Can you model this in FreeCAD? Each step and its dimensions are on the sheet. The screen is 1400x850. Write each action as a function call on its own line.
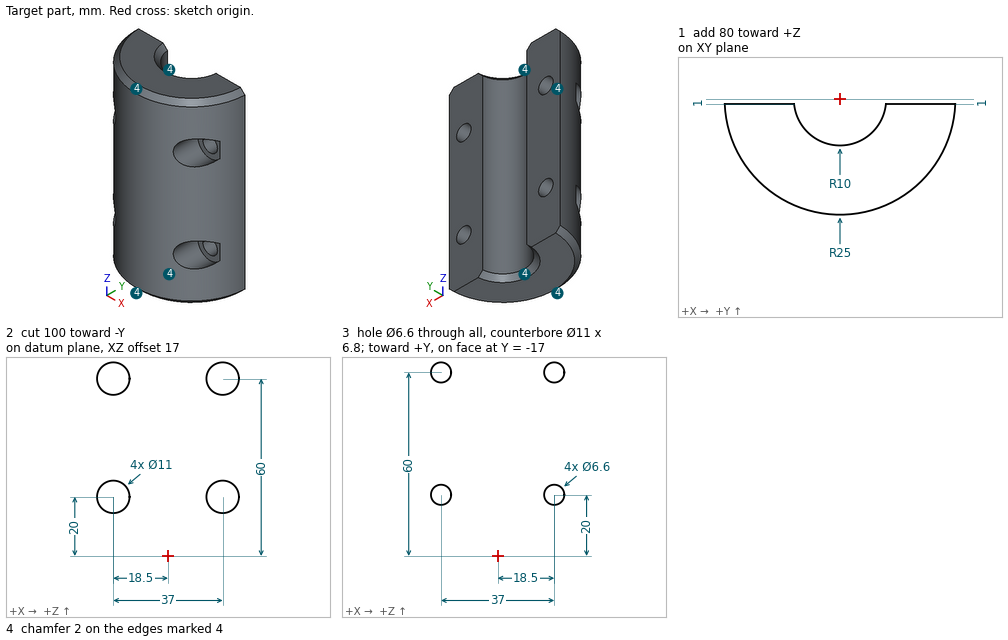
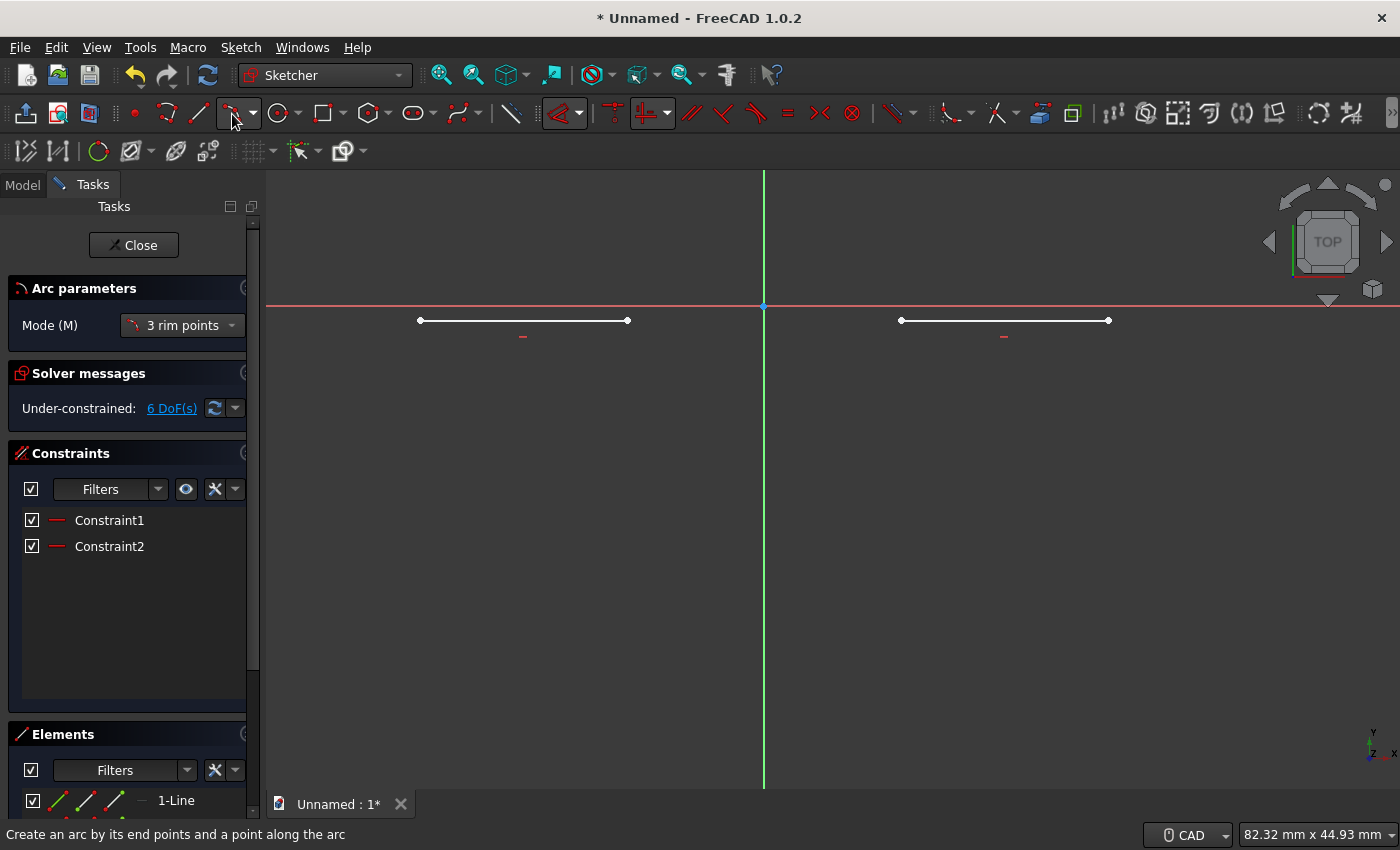
click(420, 321)
click(1108, 321)
click(660, 635)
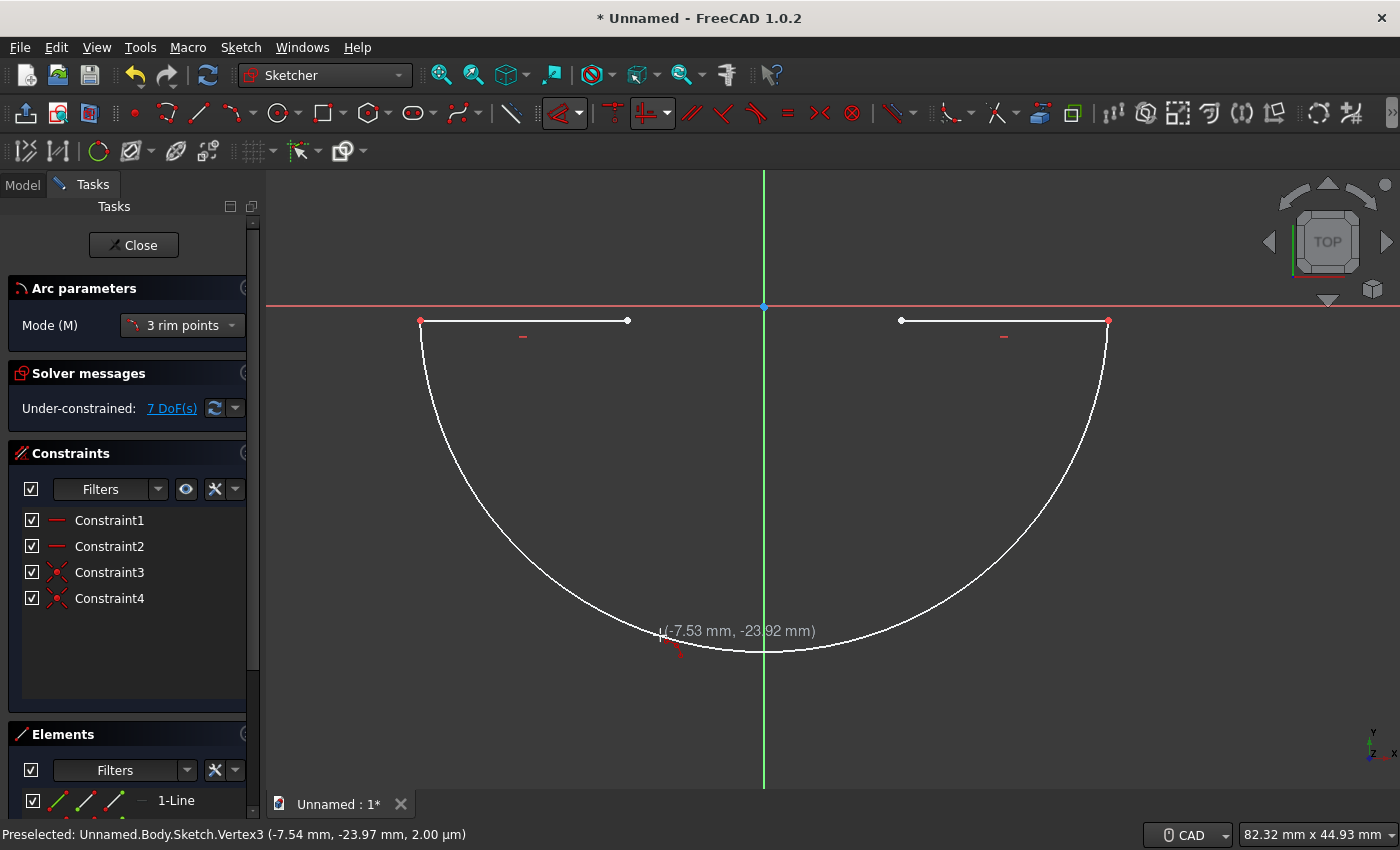
click(901, 321)
click(627, 321)
click(724, 438)
key(Escape)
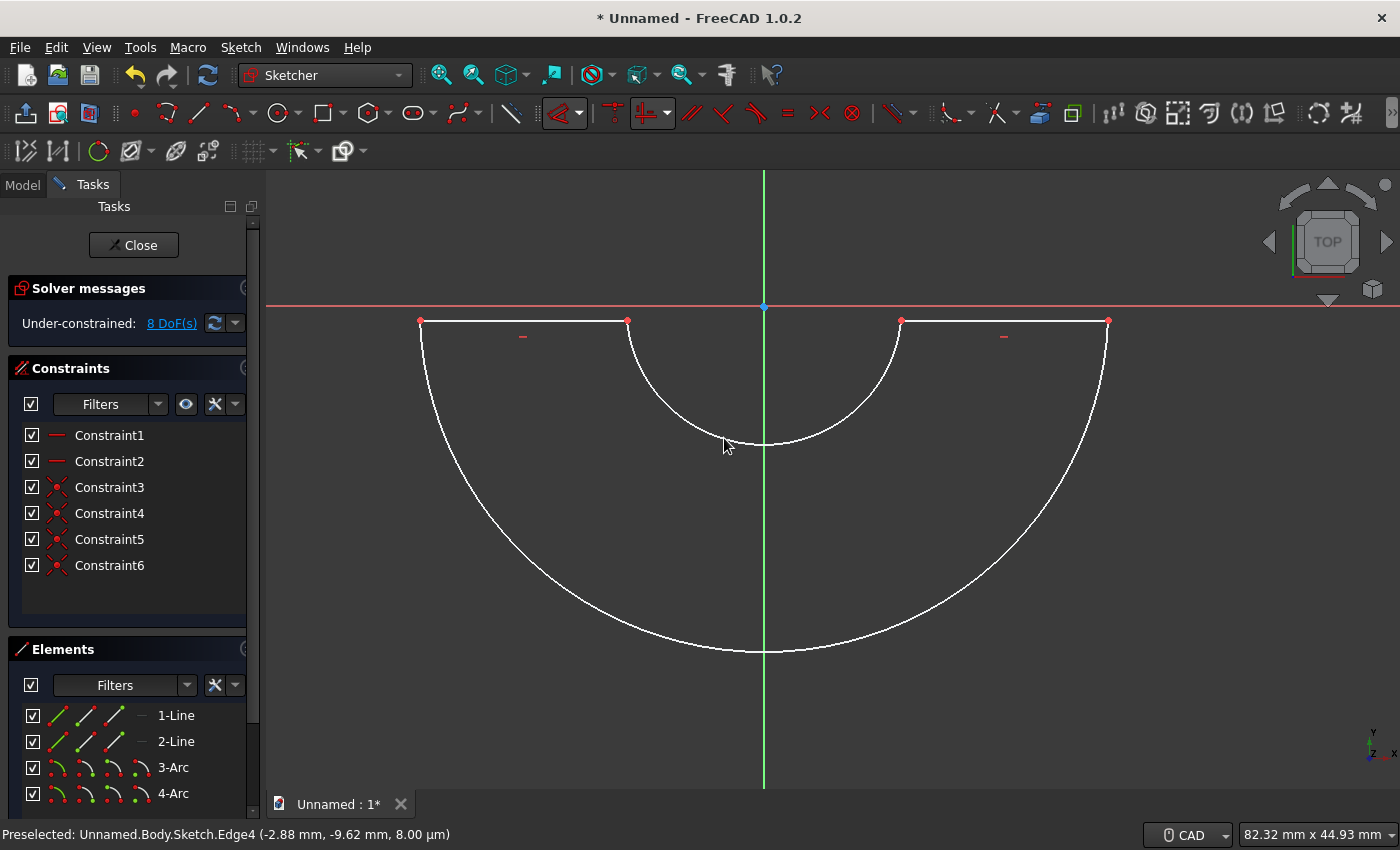
click(566, 589)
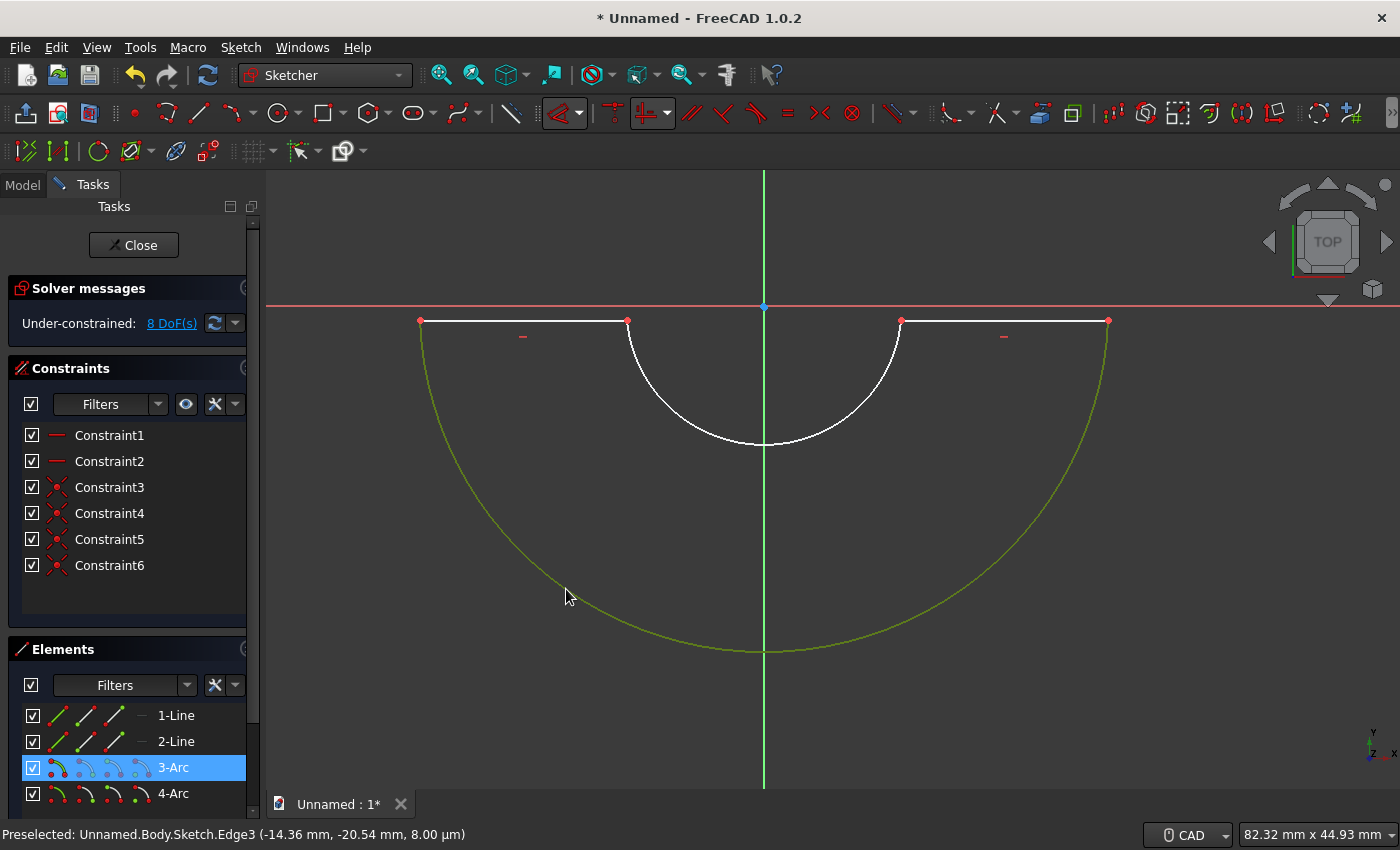
click(688, 422)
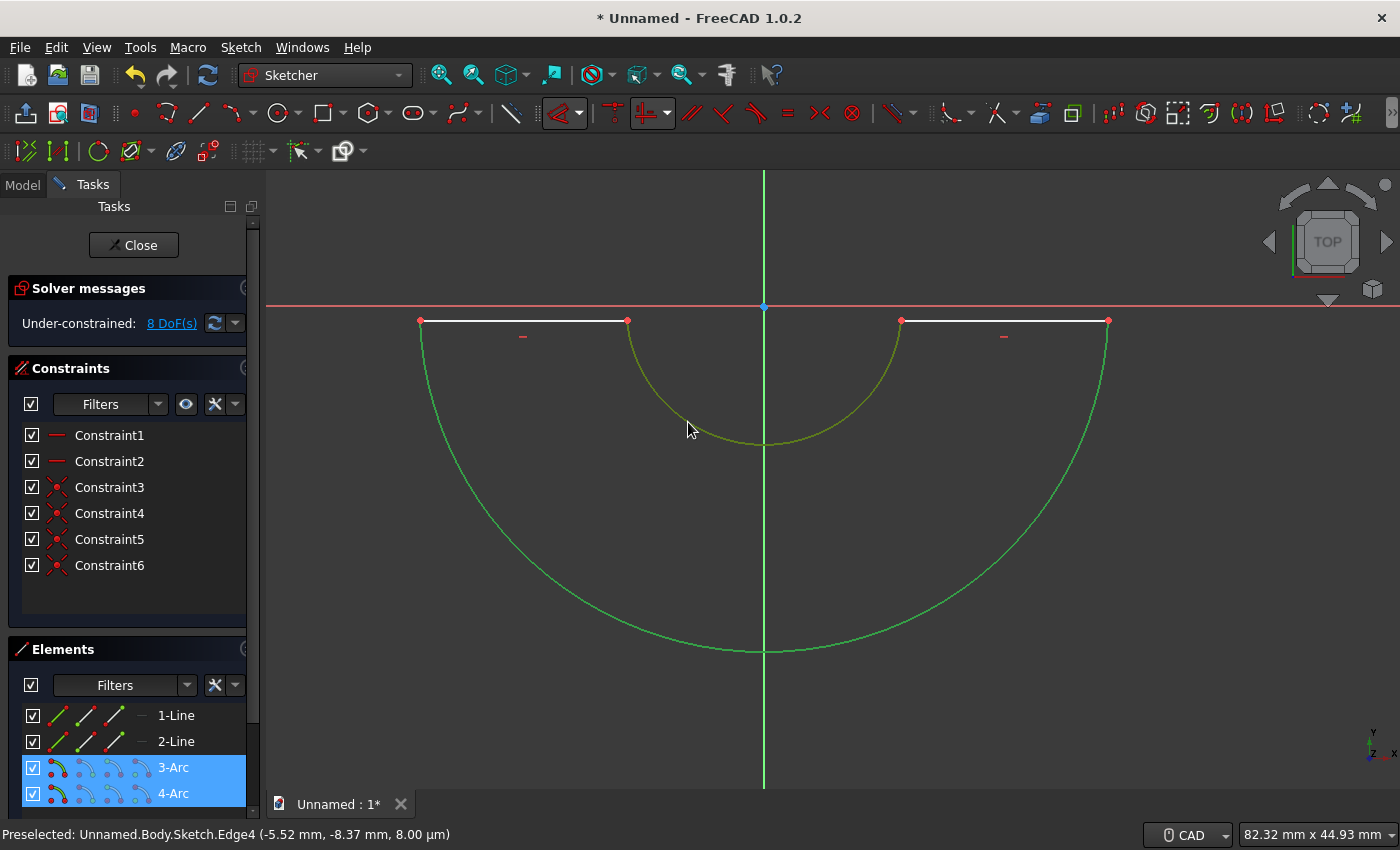
click(614, 114)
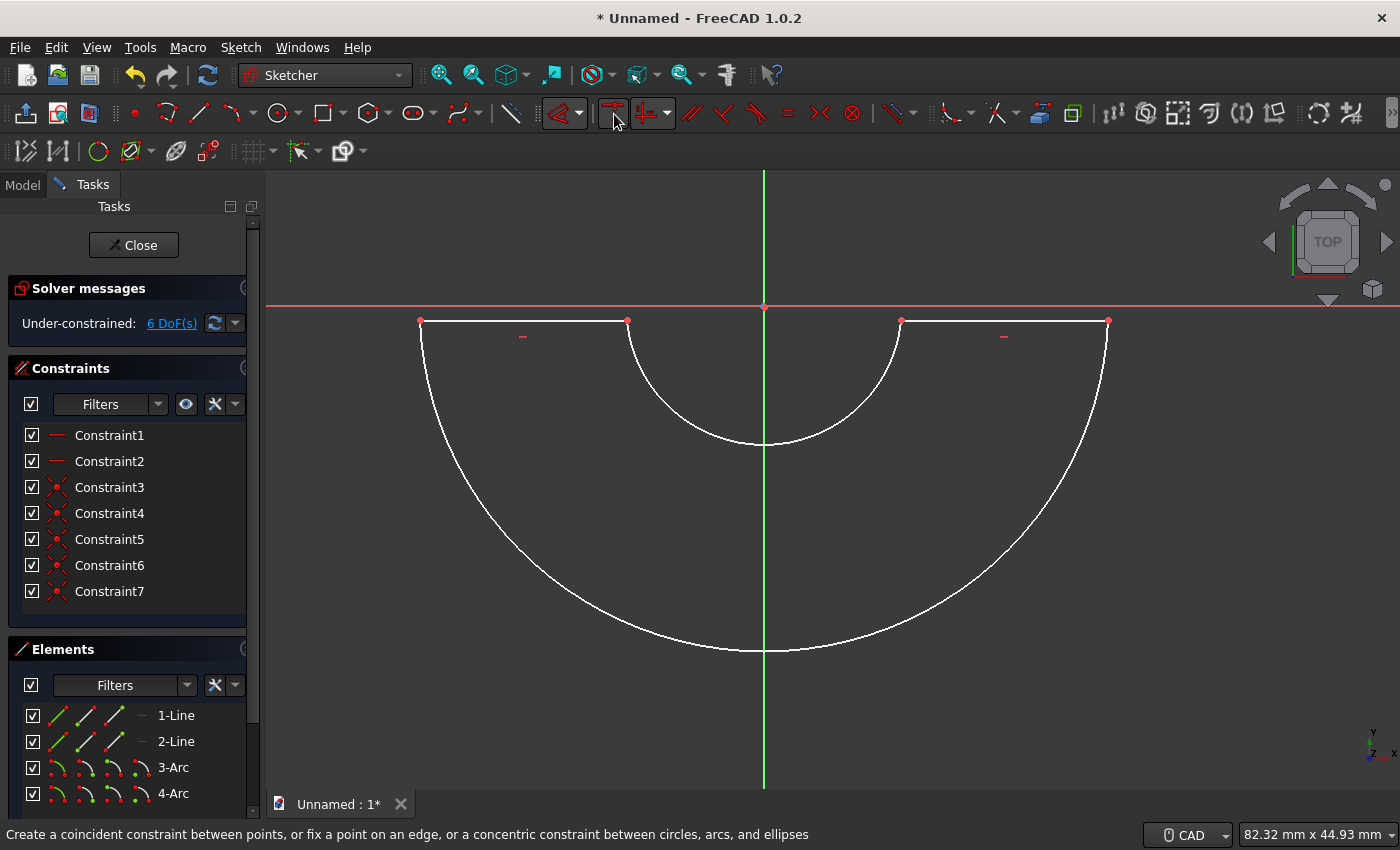
drag(754, 296, 774, 317)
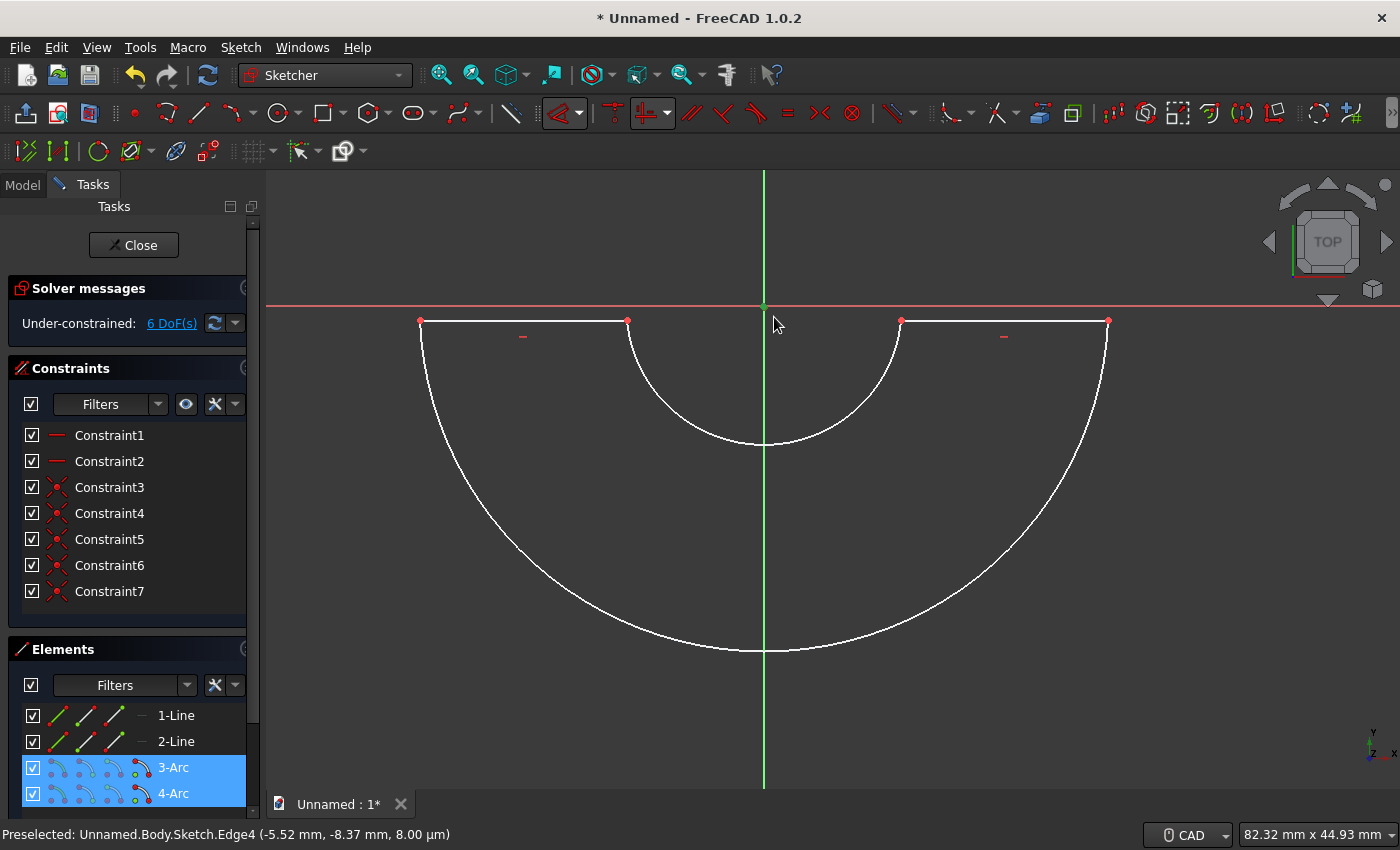
click(614, 114)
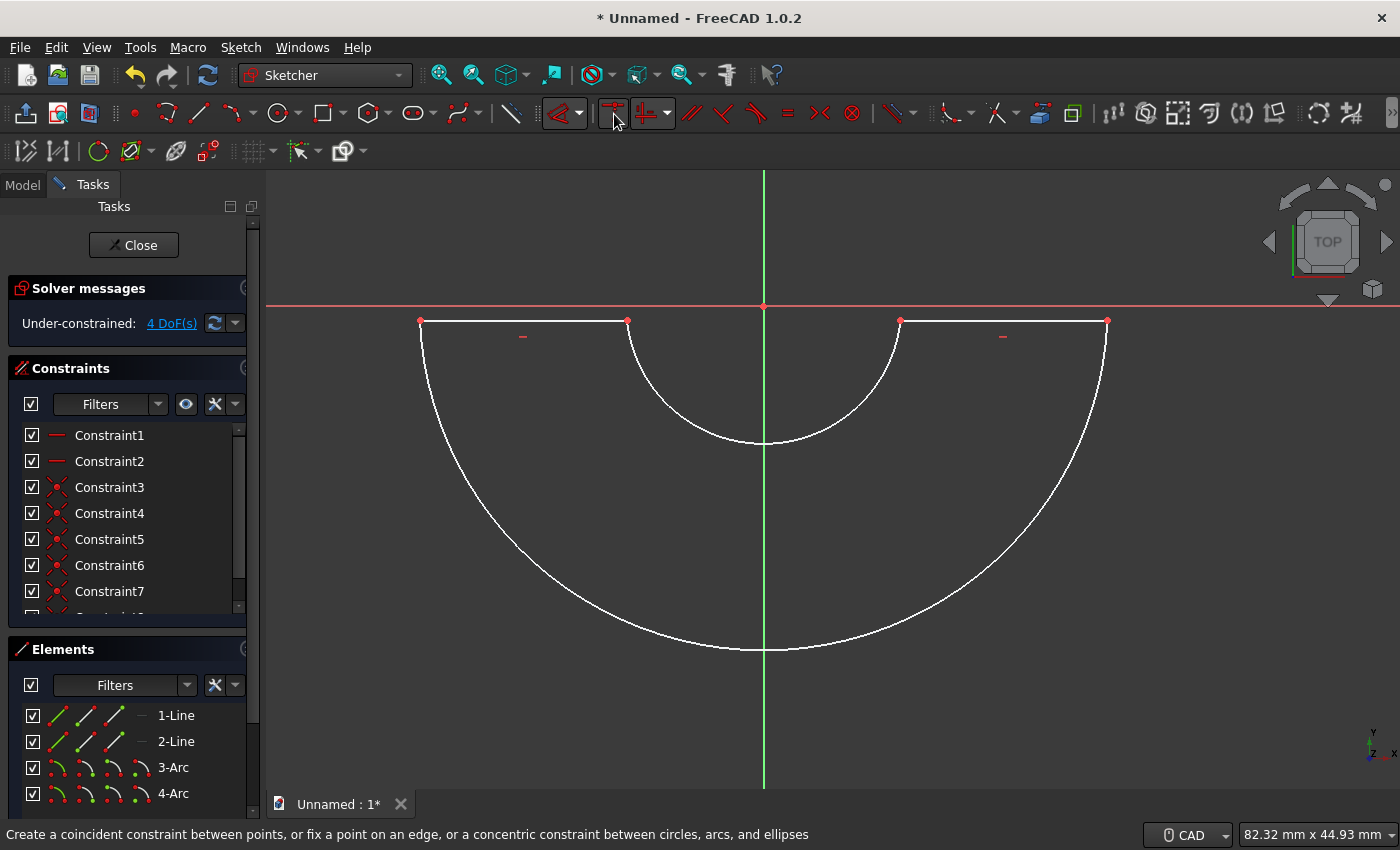
click(558, 114)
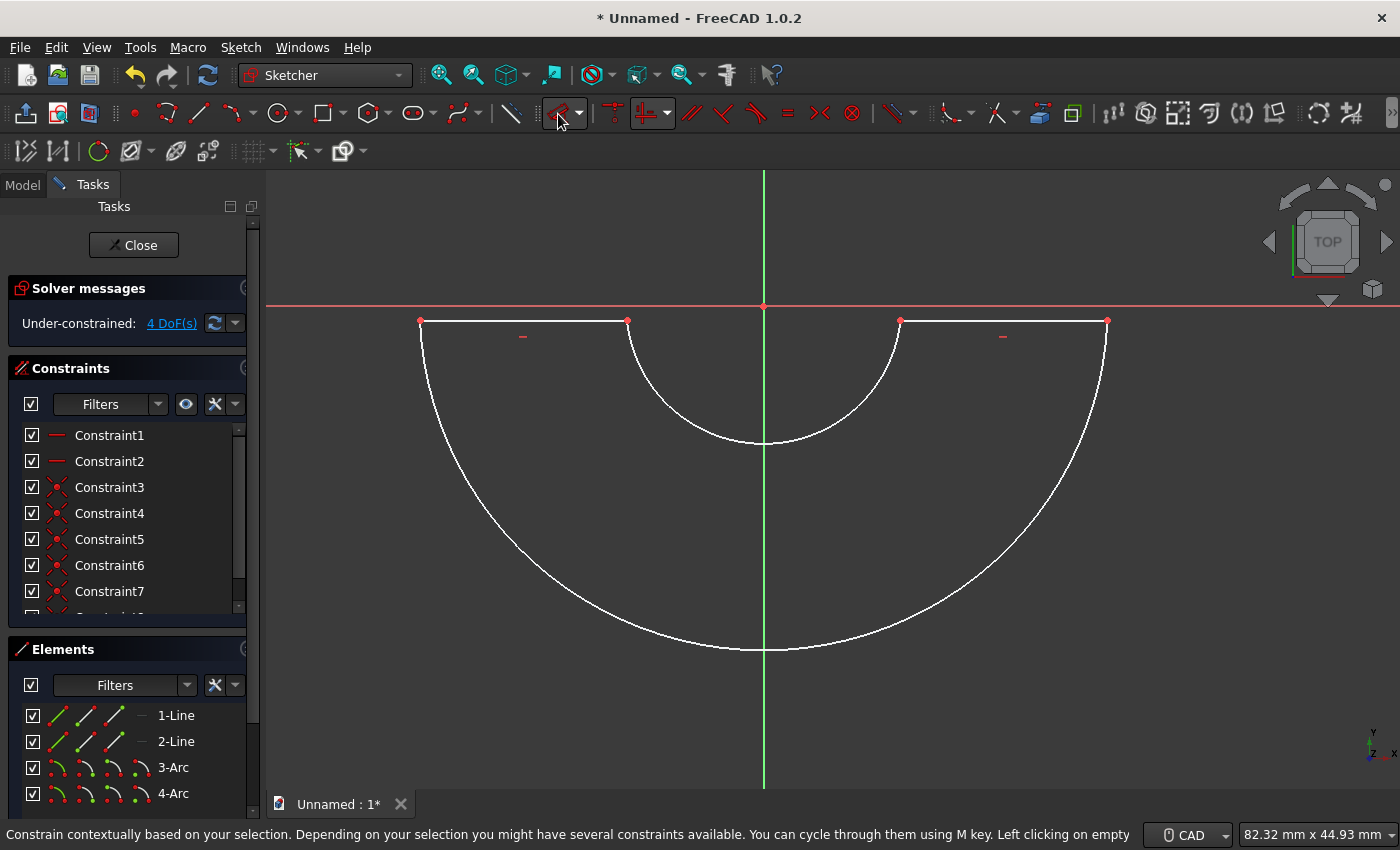
click(566, 588)
click(548, 614)